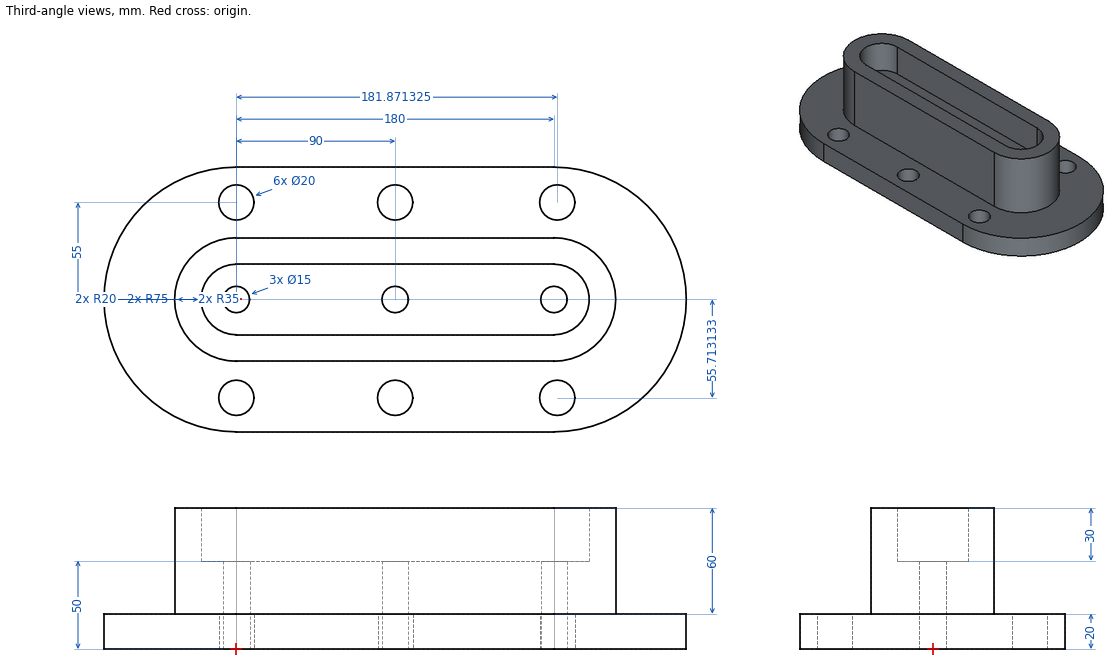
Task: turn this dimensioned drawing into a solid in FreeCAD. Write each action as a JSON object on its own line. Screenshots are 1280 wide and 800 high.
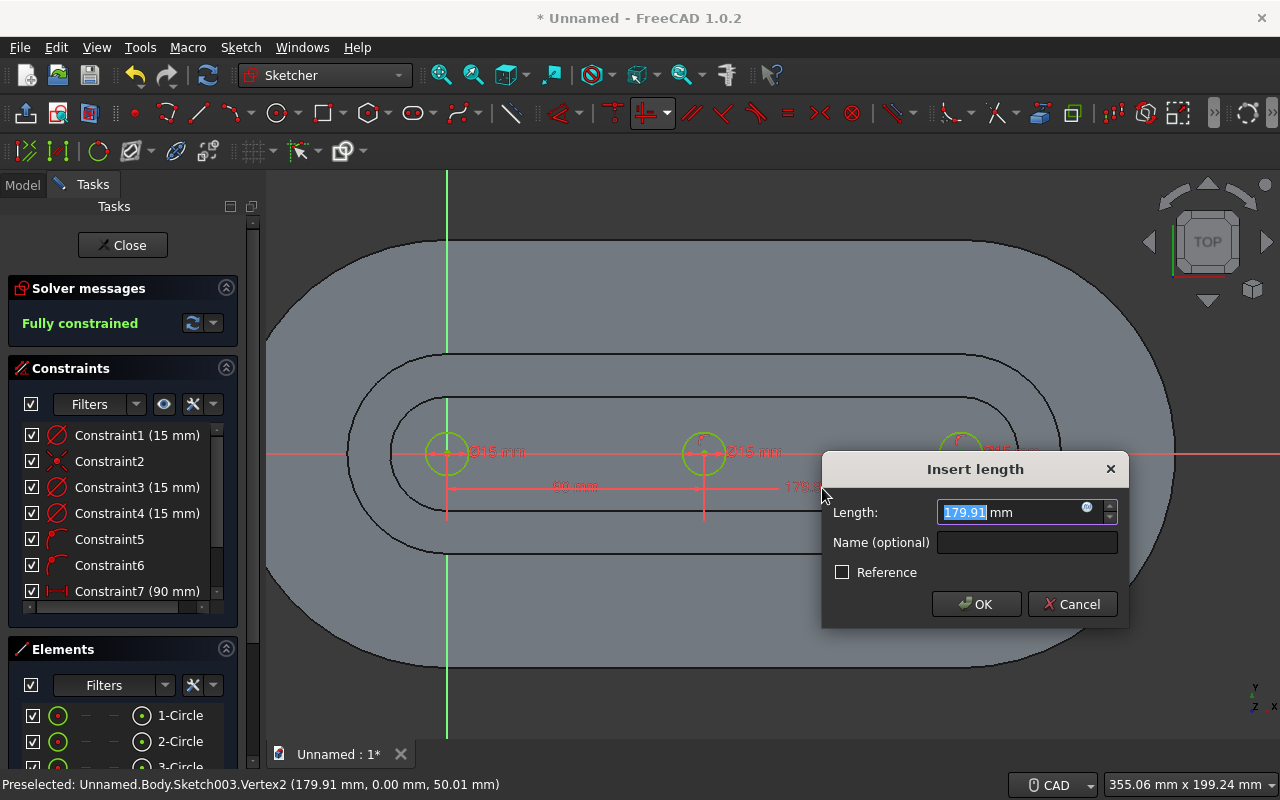
{"action": "type", "text": "180"}
{"action": "key", "text": "Return"}
{"action": "key", "text": "Escape"}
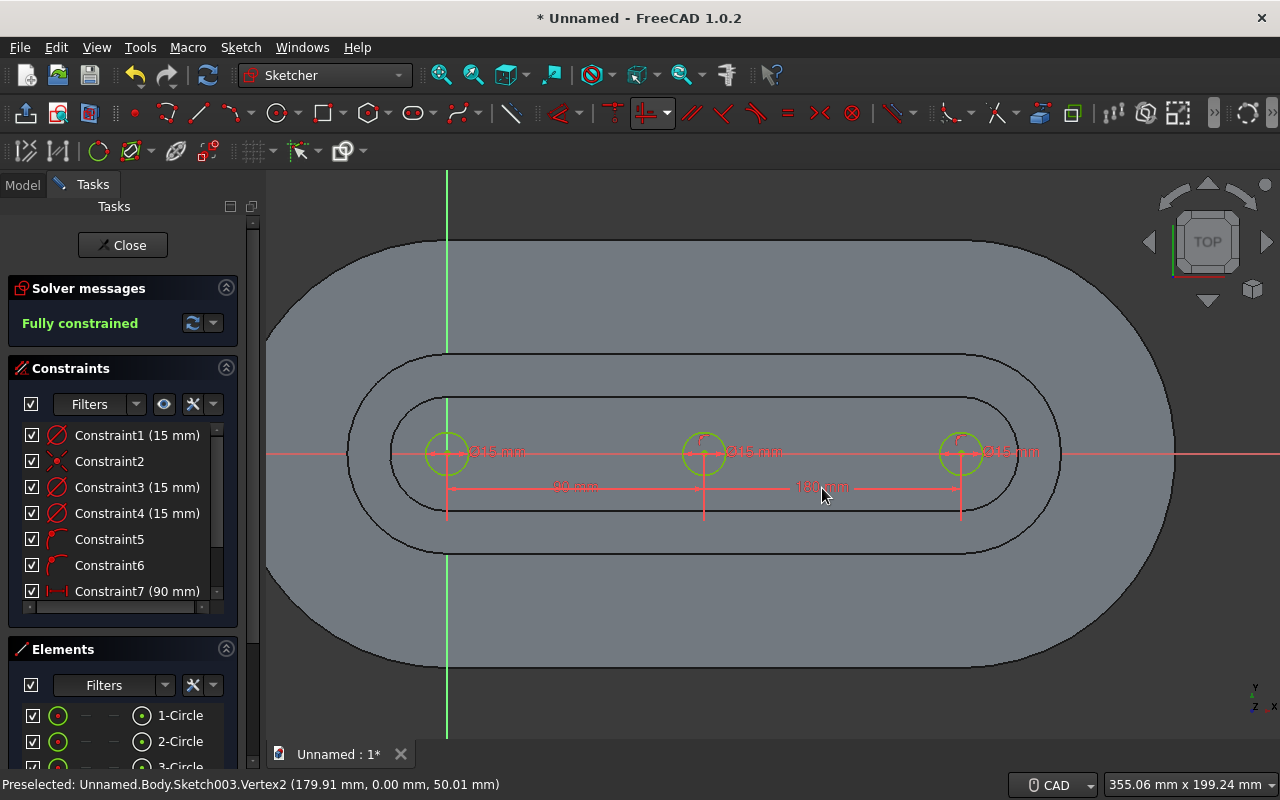
{"action": "left_click", "coordinate": [123, 245]}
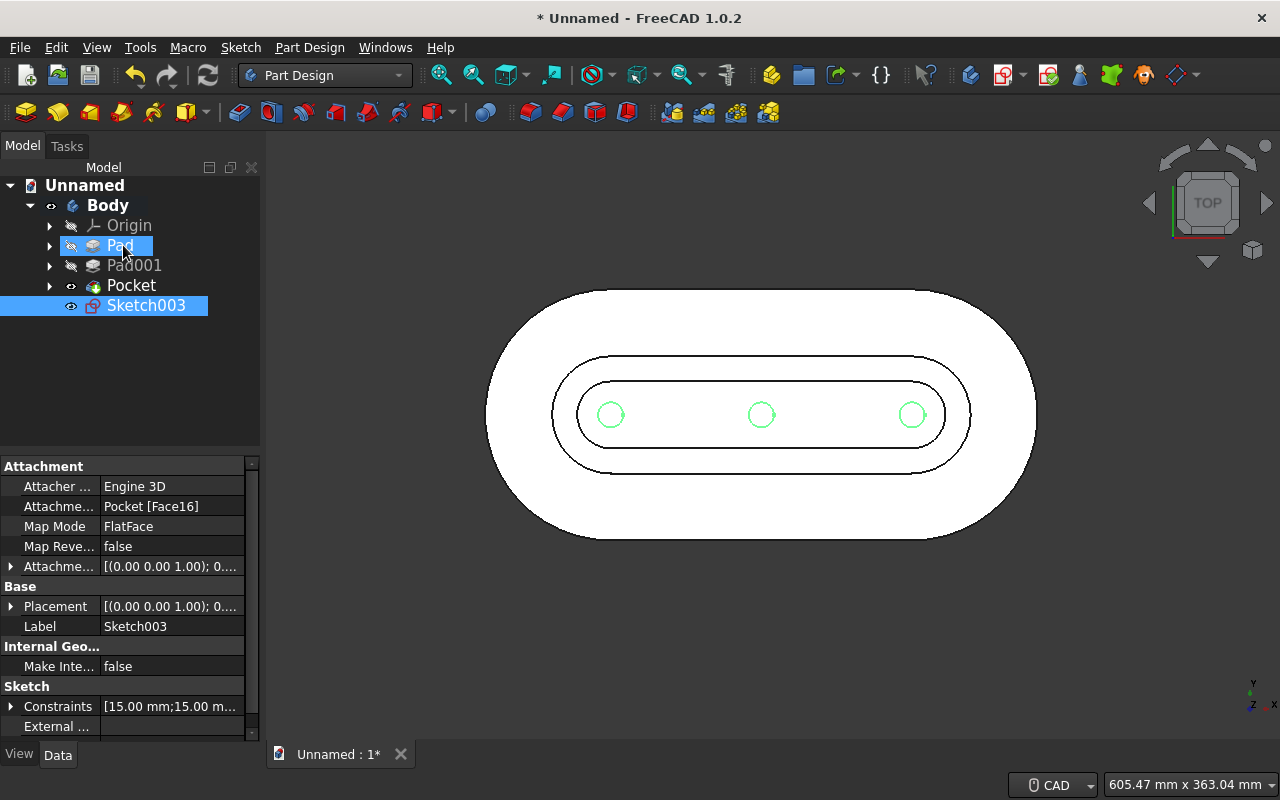
{"action": "left_click", "coordinate": [240, 112]}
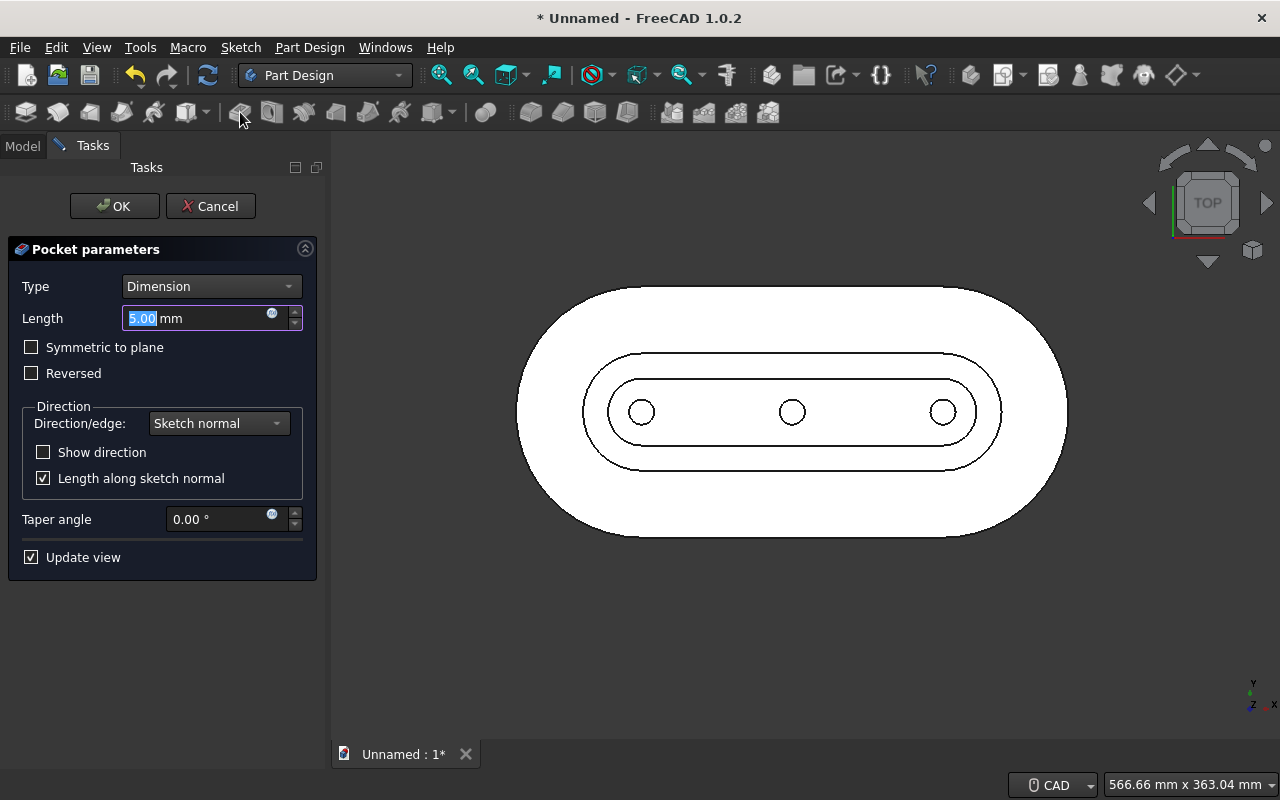
{"action": "type", "text": "50"}
{"action": "key", "text": "Tab"}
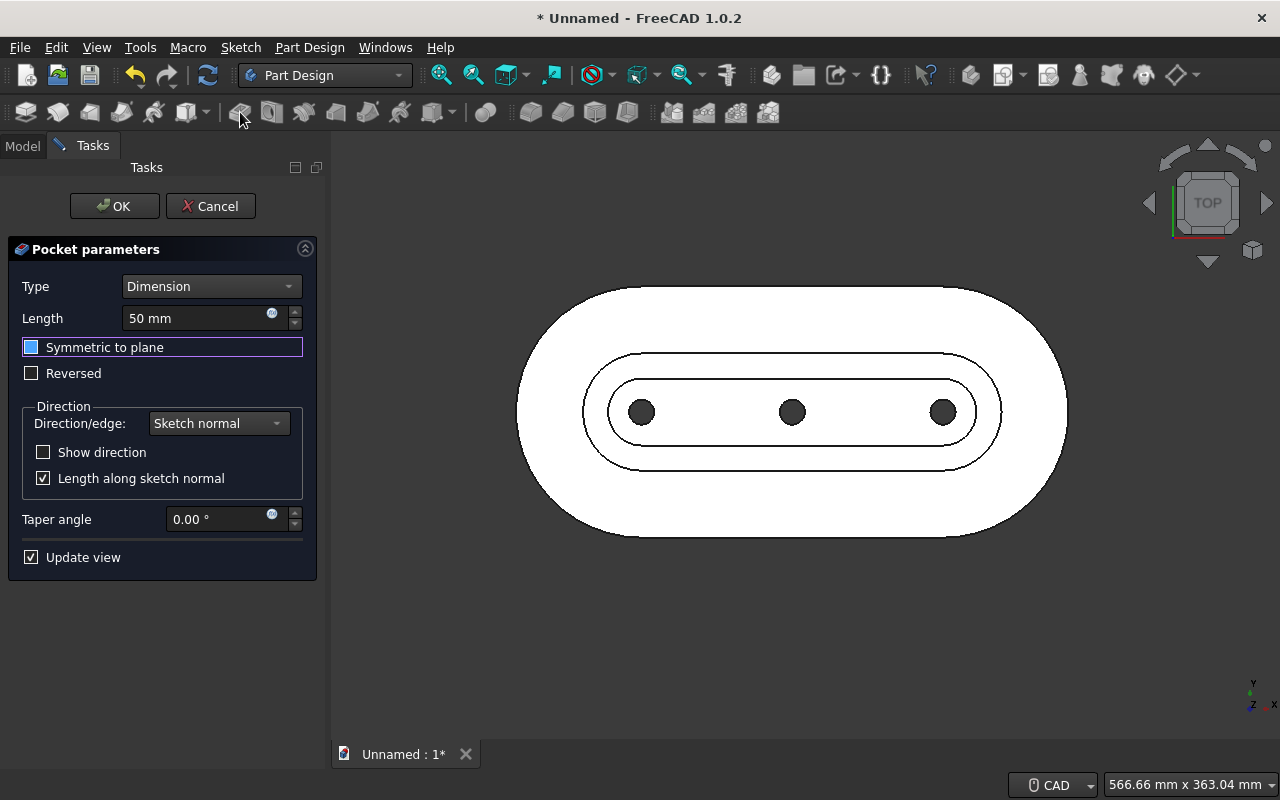
{"action": "left_click", "coordinate": [115, 206]}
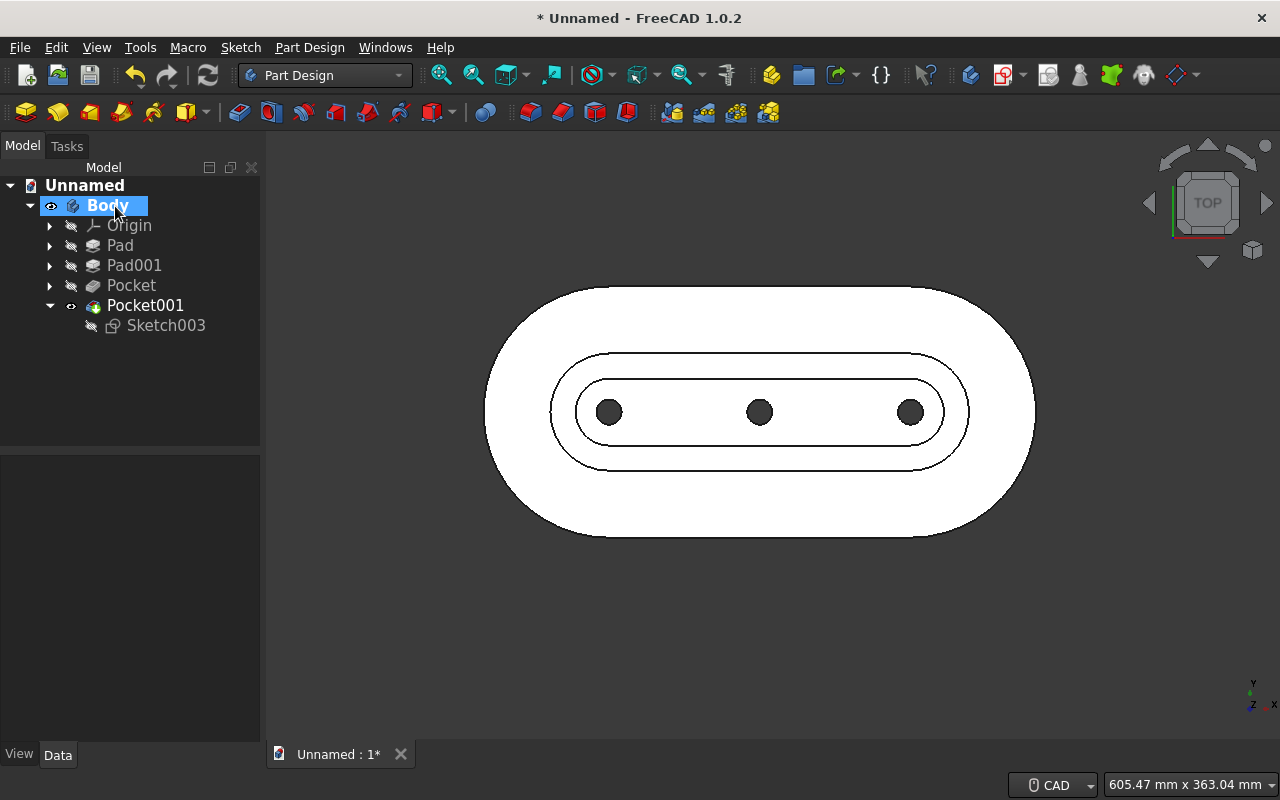
{"action": "left_click", "coordinate": [523, 375]}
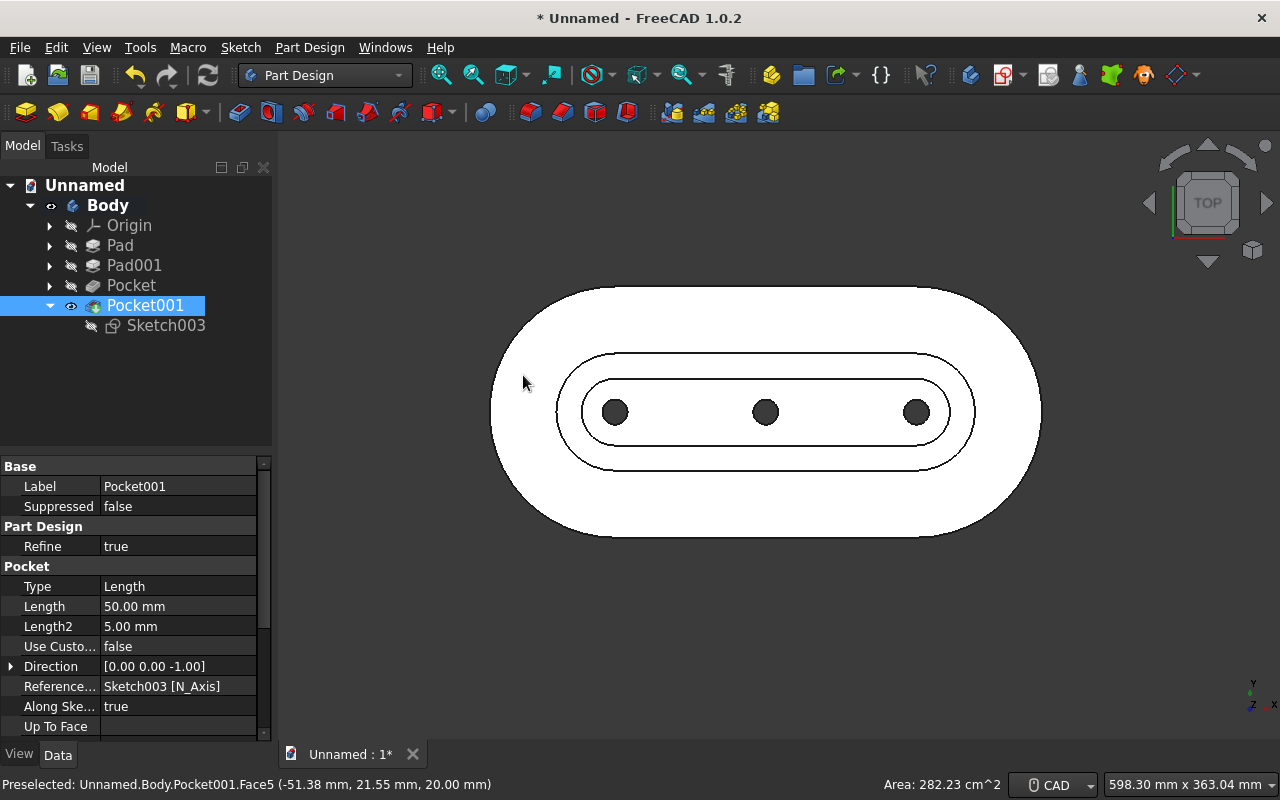
{"action": "left_click", "coordinate": [1004, 76]}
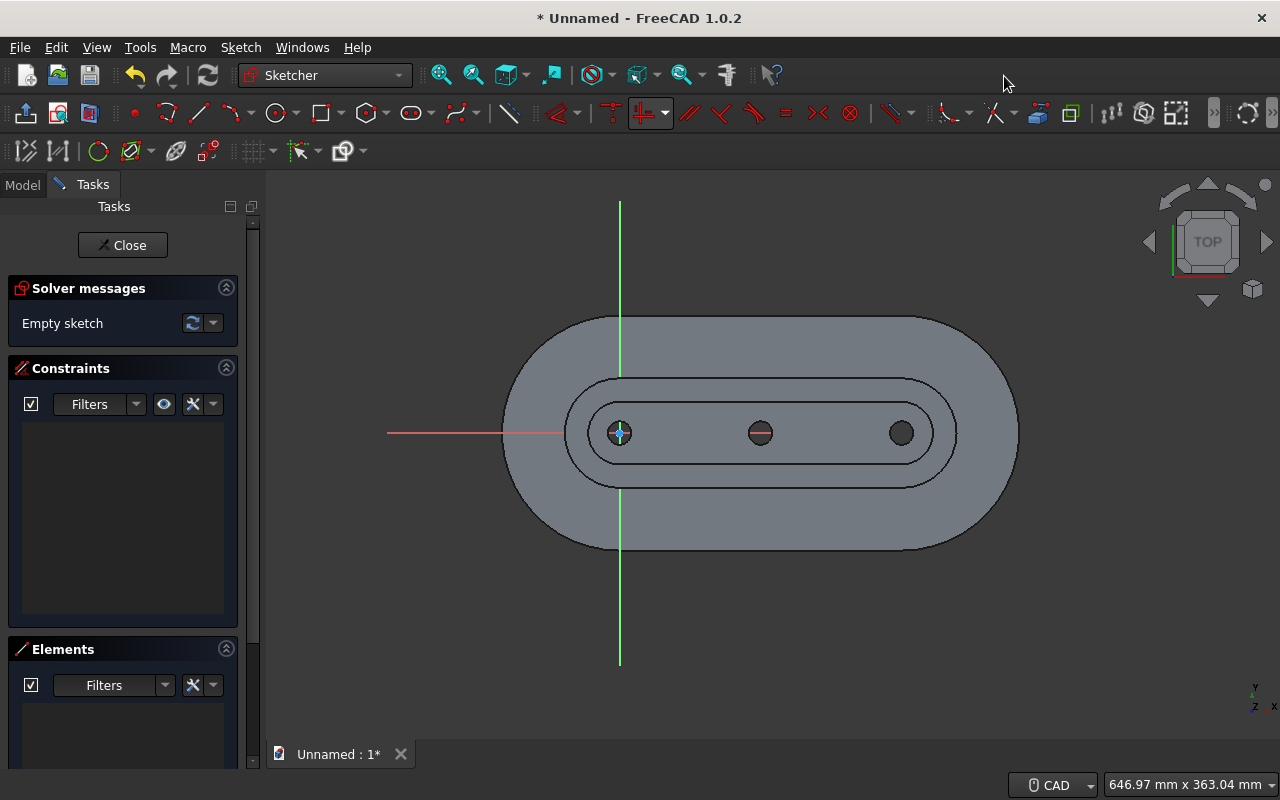
{"action": "scroll", "coordinate": [832, 408], "scroll_direction": "up", "scroll_amount": 3}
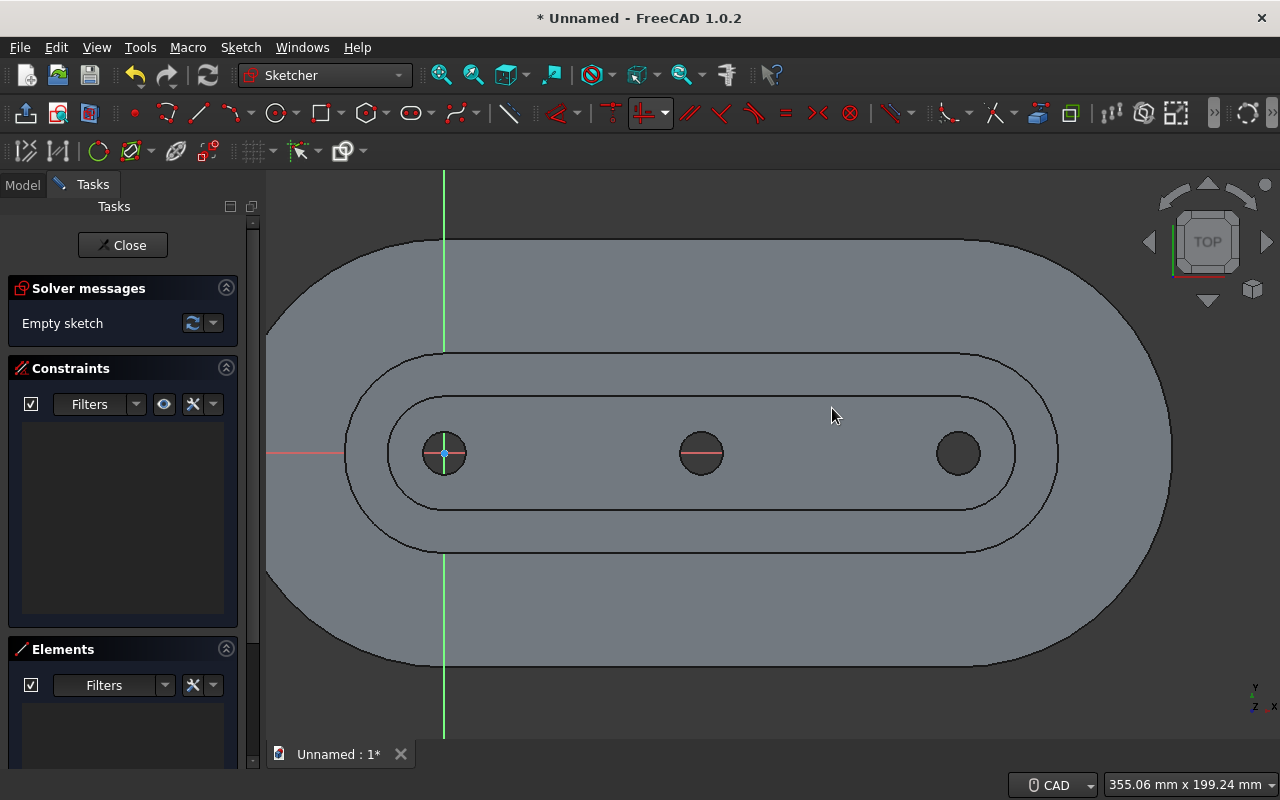
{"action": "left_click", "coordinate": [276, 114]}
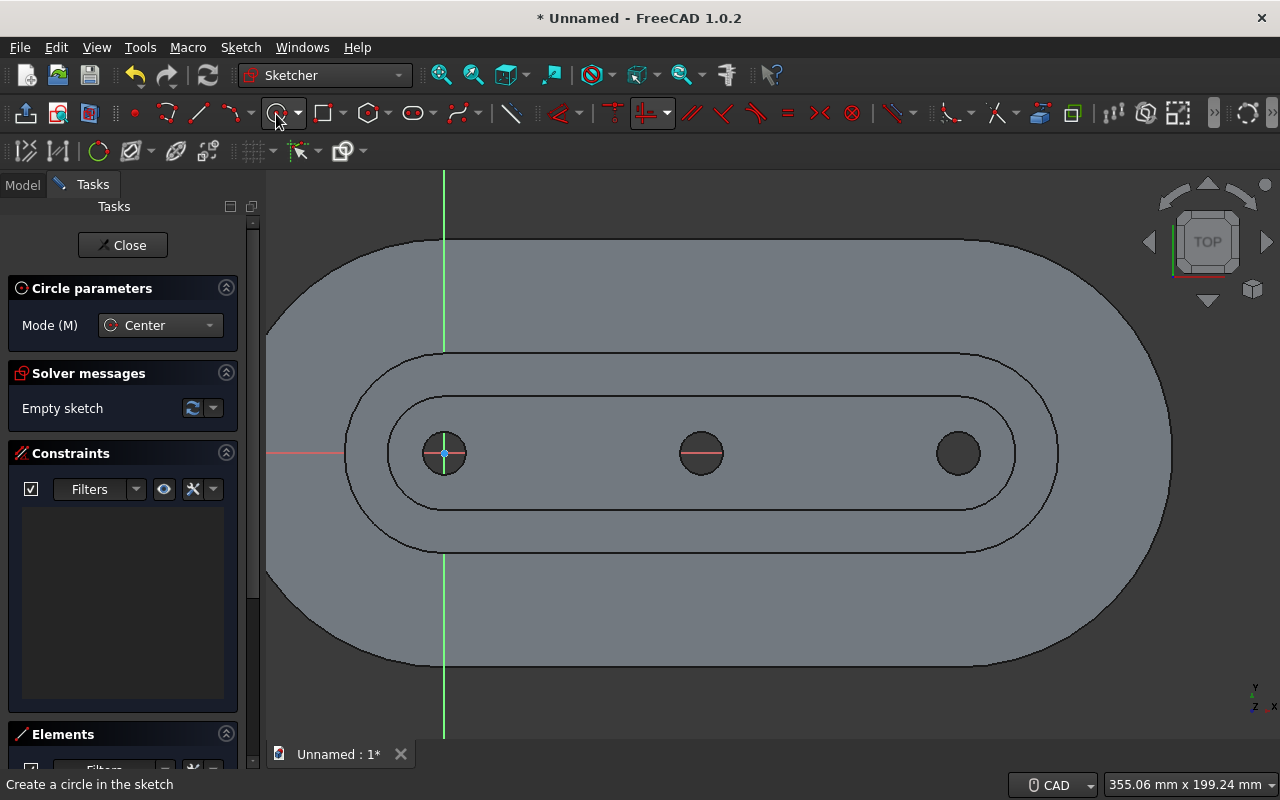
{"action": "left_click", "coordinate": [444, 296]}
{"action": "mouse_move", "coordinate": [465, 276]}